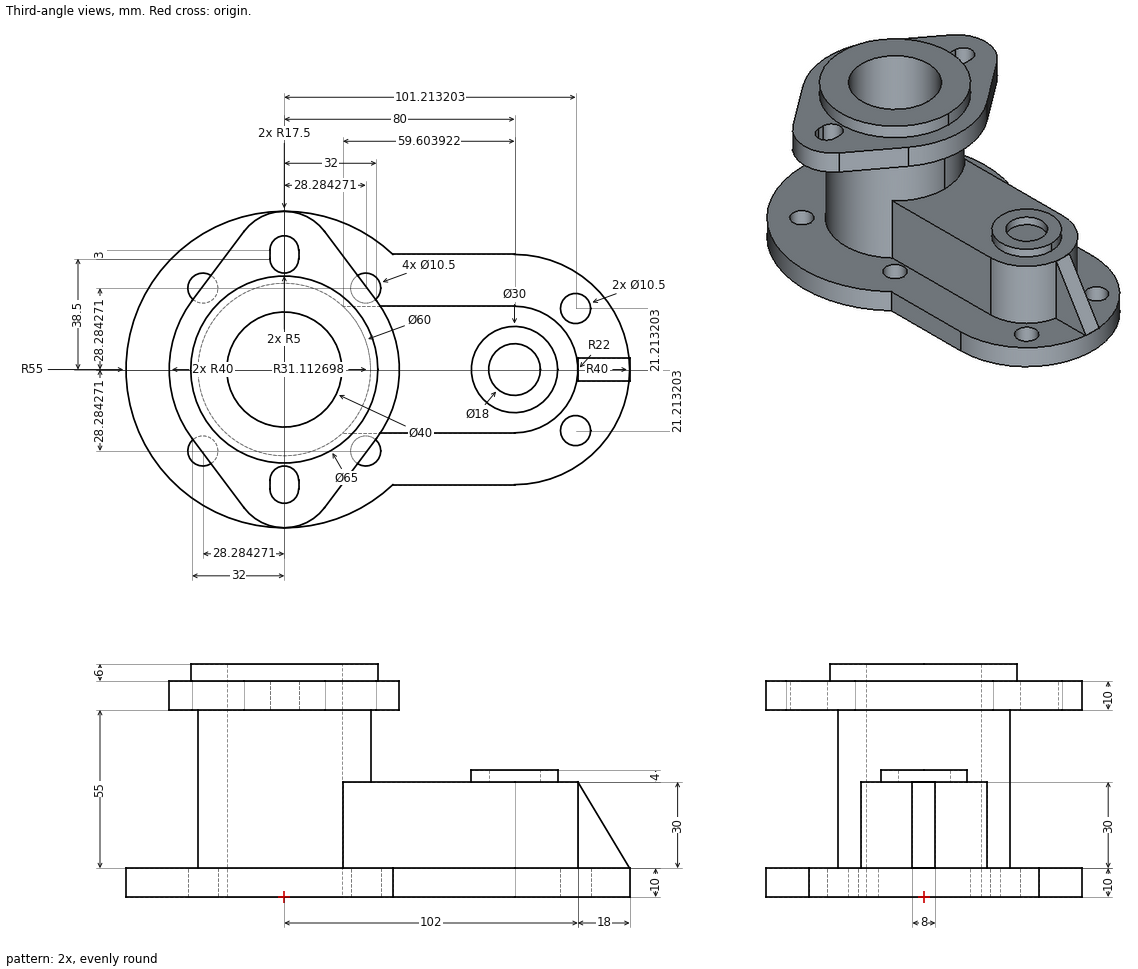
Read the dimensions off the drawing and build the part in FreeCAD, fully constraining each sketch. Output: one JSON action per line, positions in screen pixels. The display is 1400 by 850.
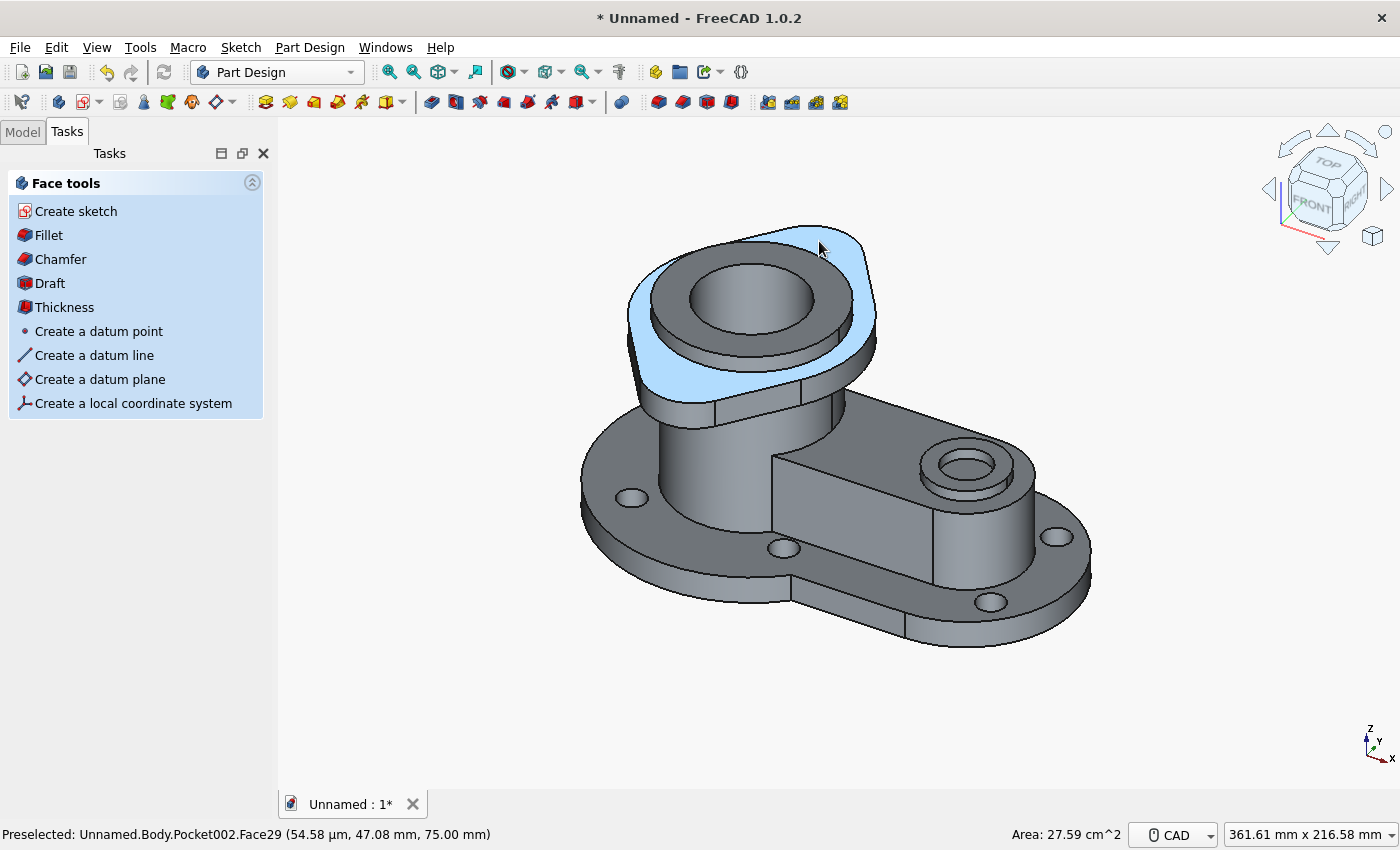
{"action": "left_click", "coordinate": [84, 102]}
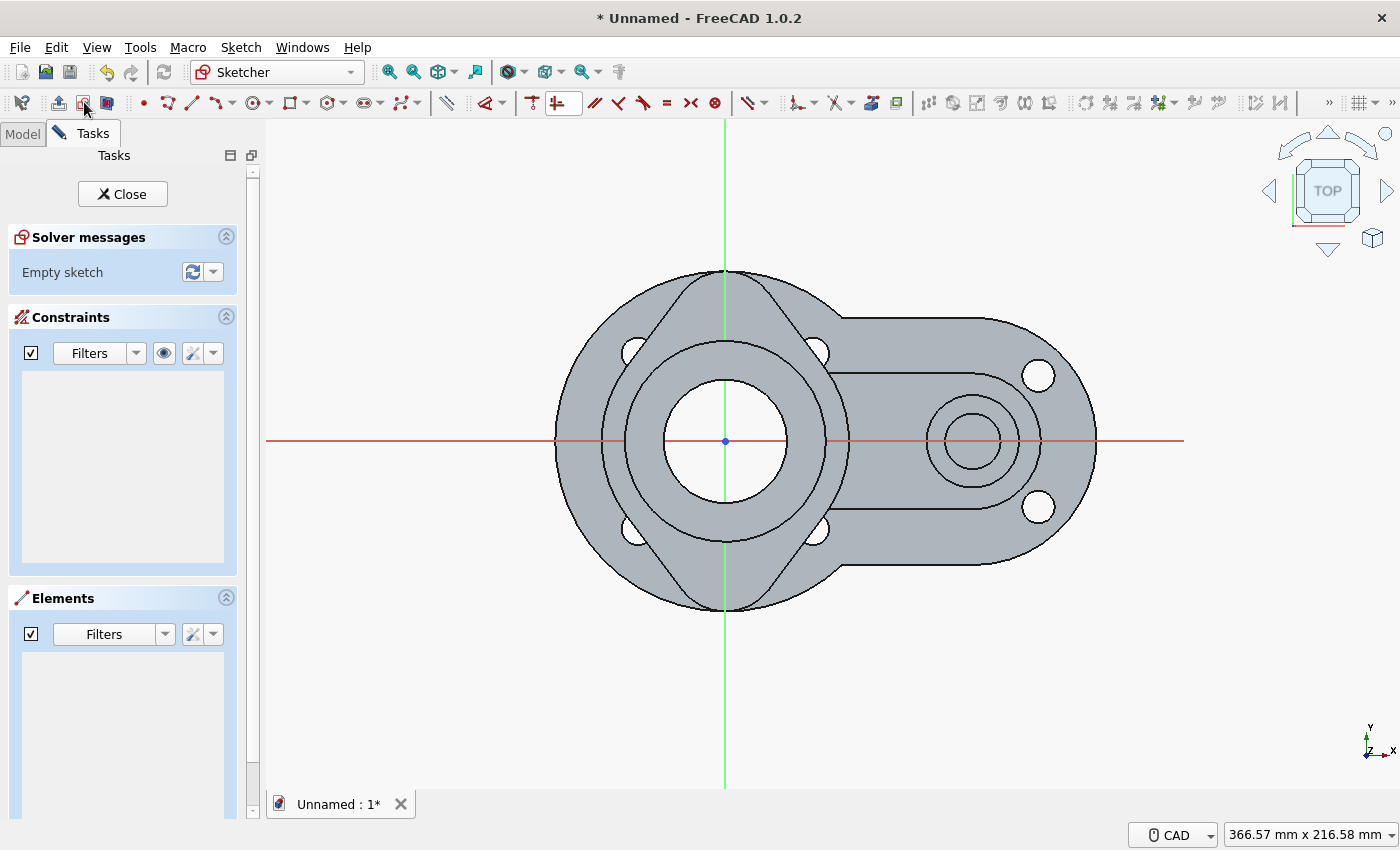
{"action": "key", "text": "q s"}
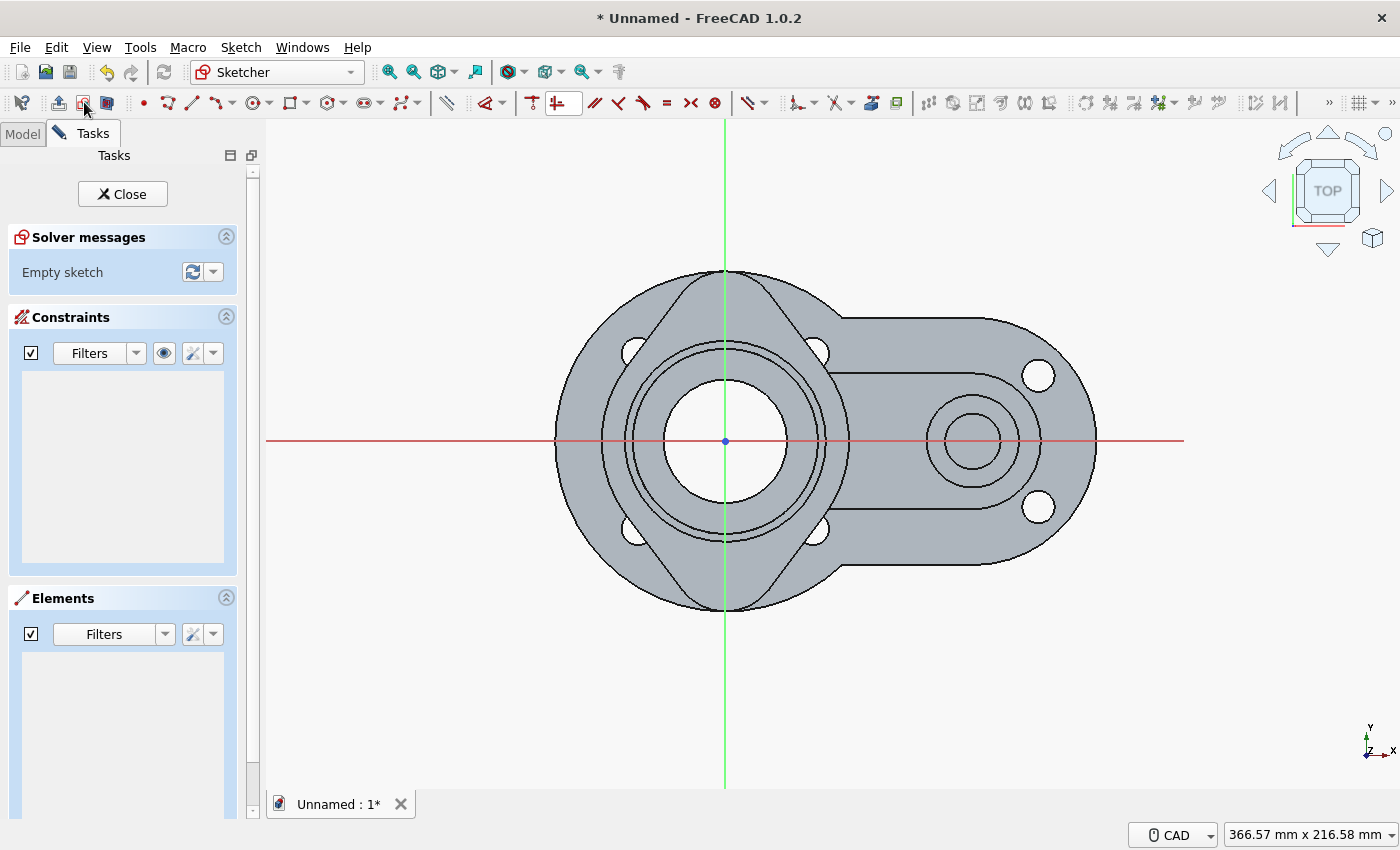
{"action": "scroll", "coordinate": [721, 304], "scroll_direction": "up", "scroll_amount": 12}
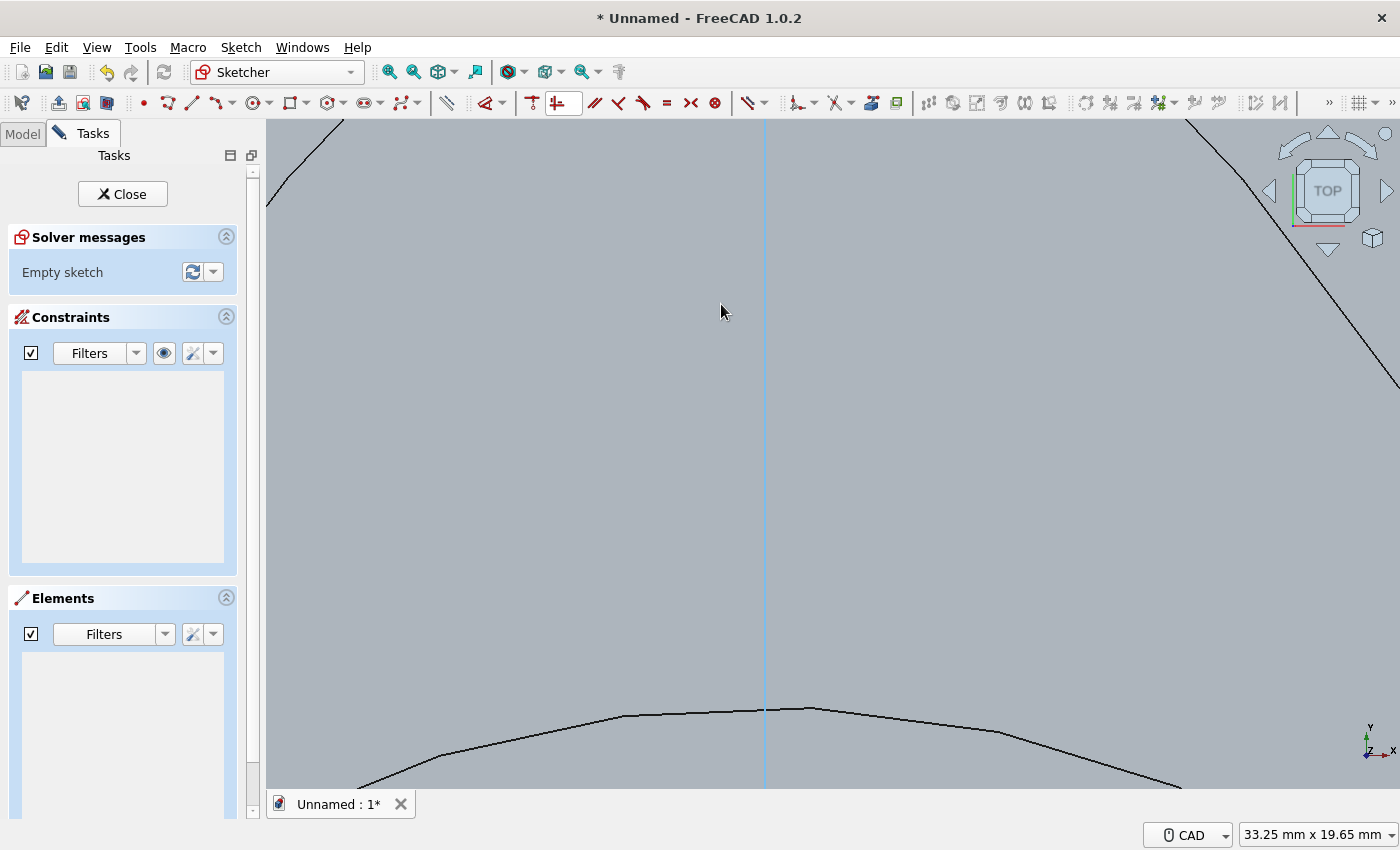
{"action": "key", "text": "g s"}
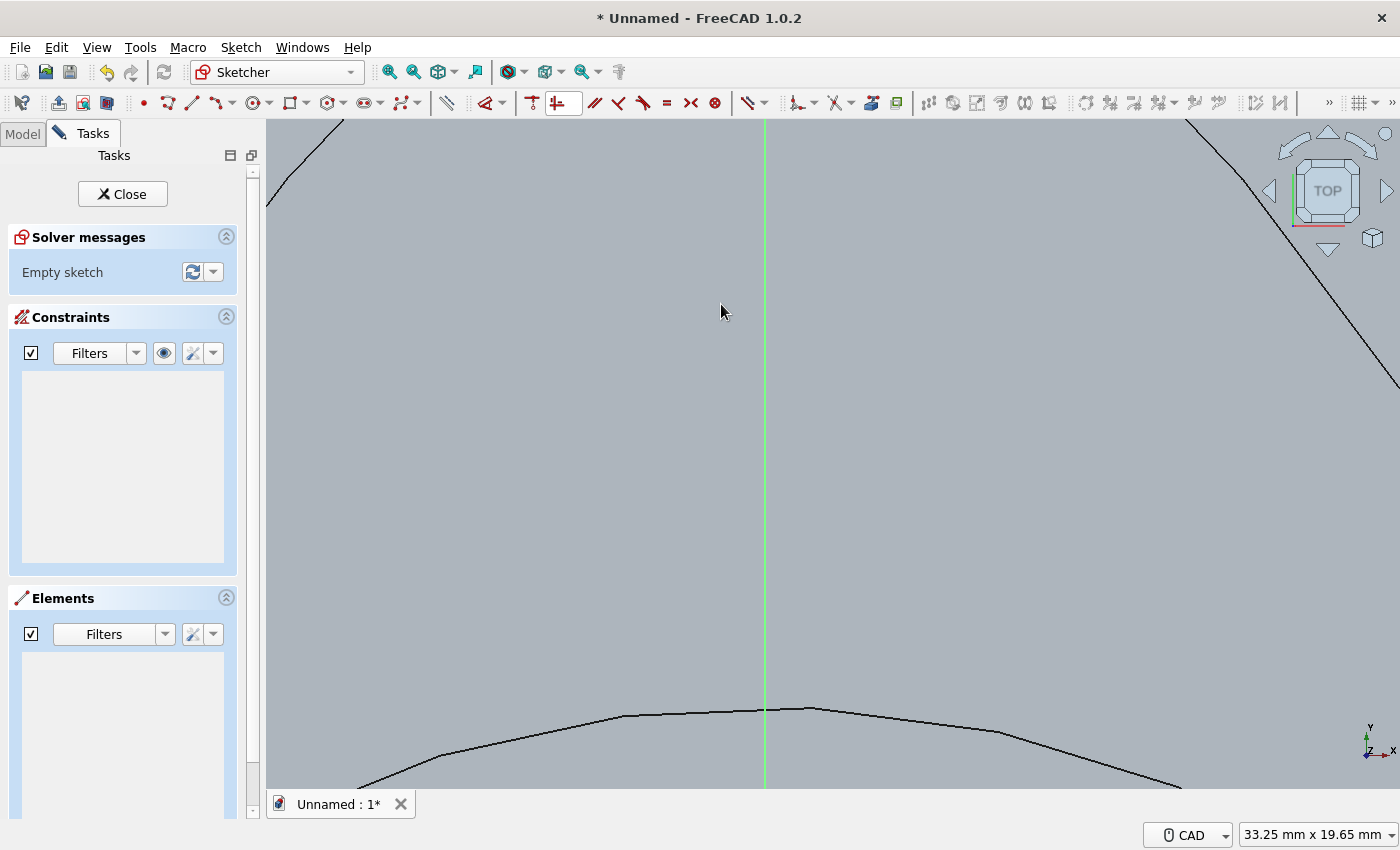
{"action": "left_click", "coordinate": [765, 503]}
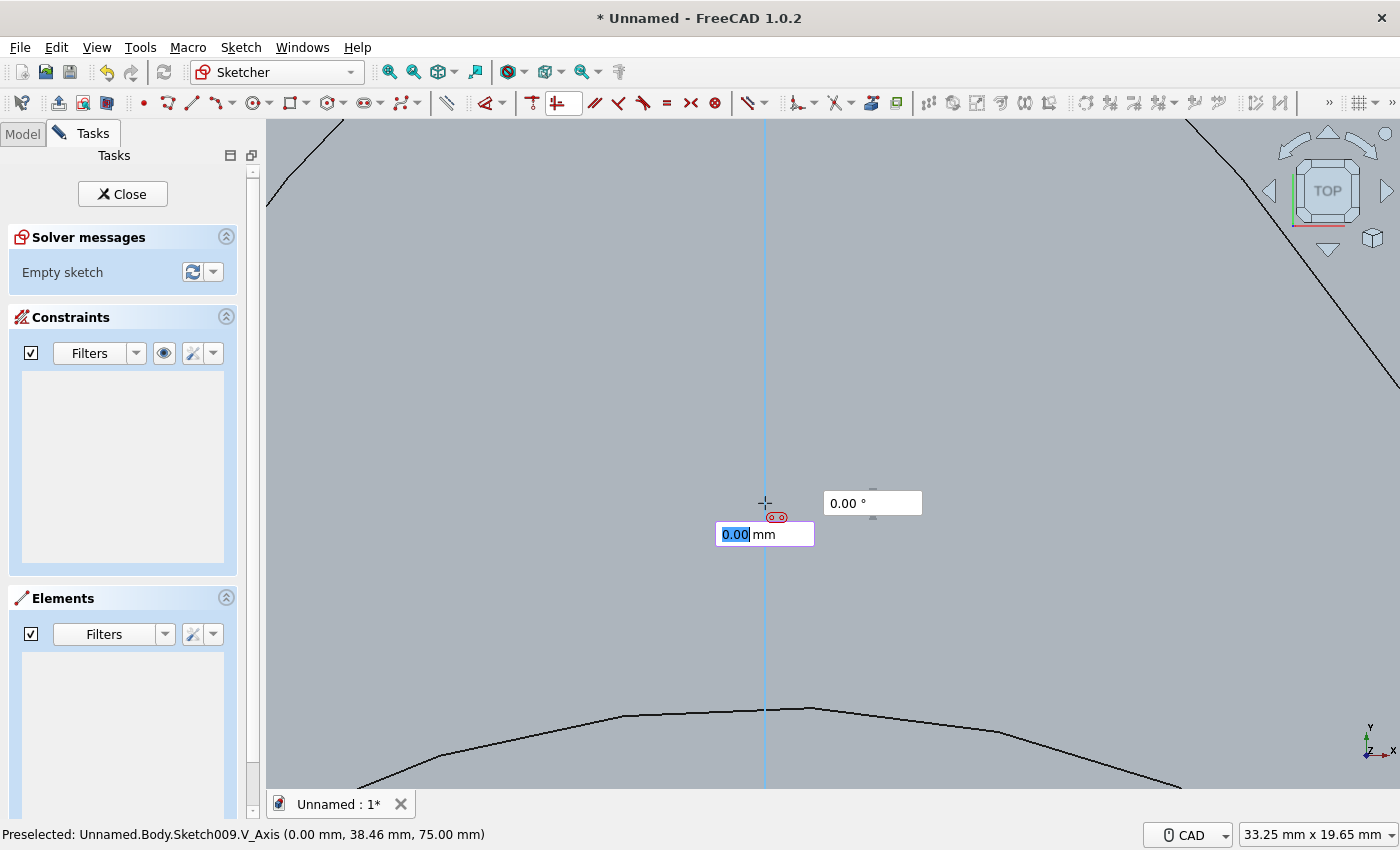
{"action": "left_click", "coordinate": [774, 400]}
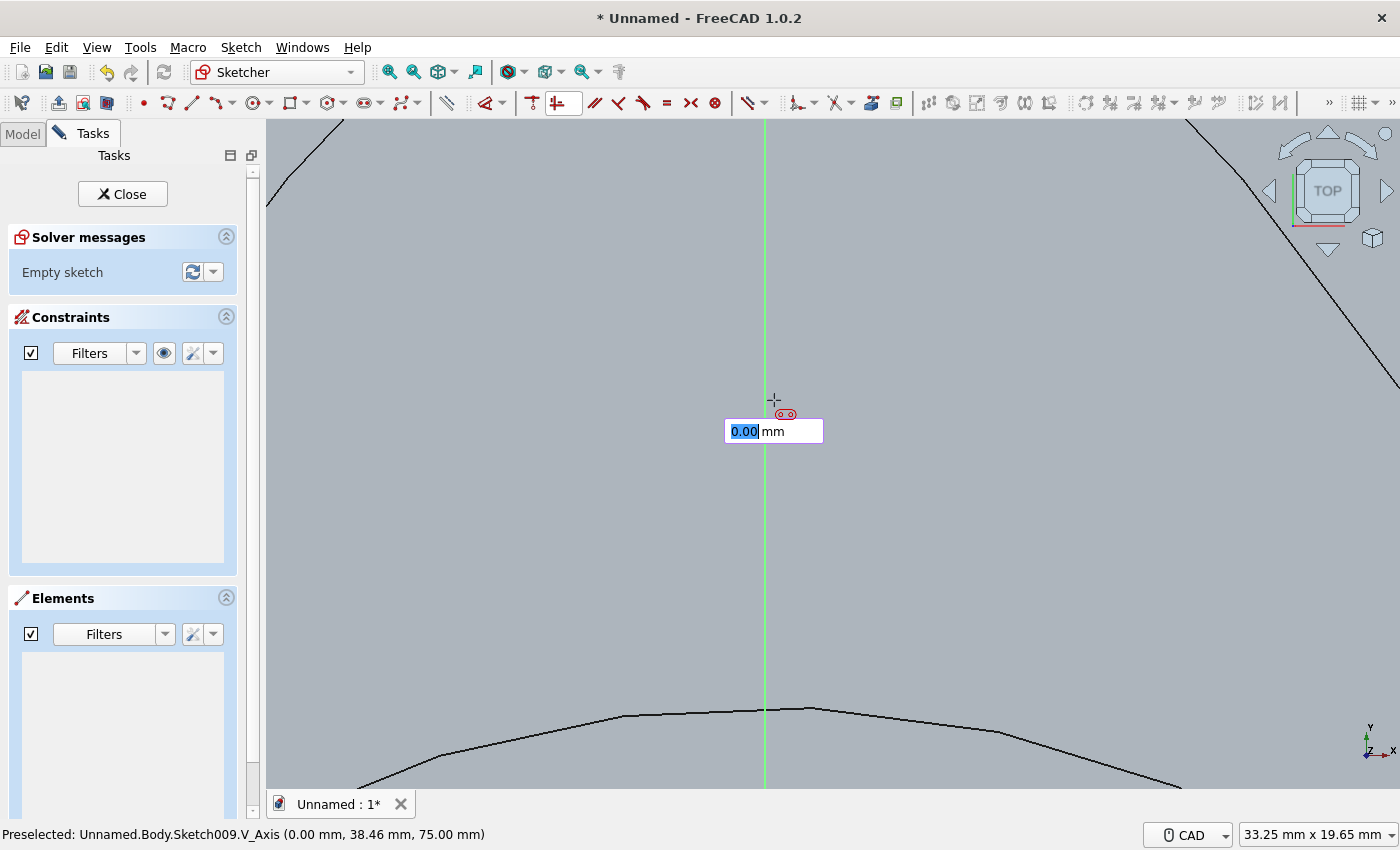
{"action": "left_click", "coordinate": [594, 451]}
{"action": "key", "text": "Escape"}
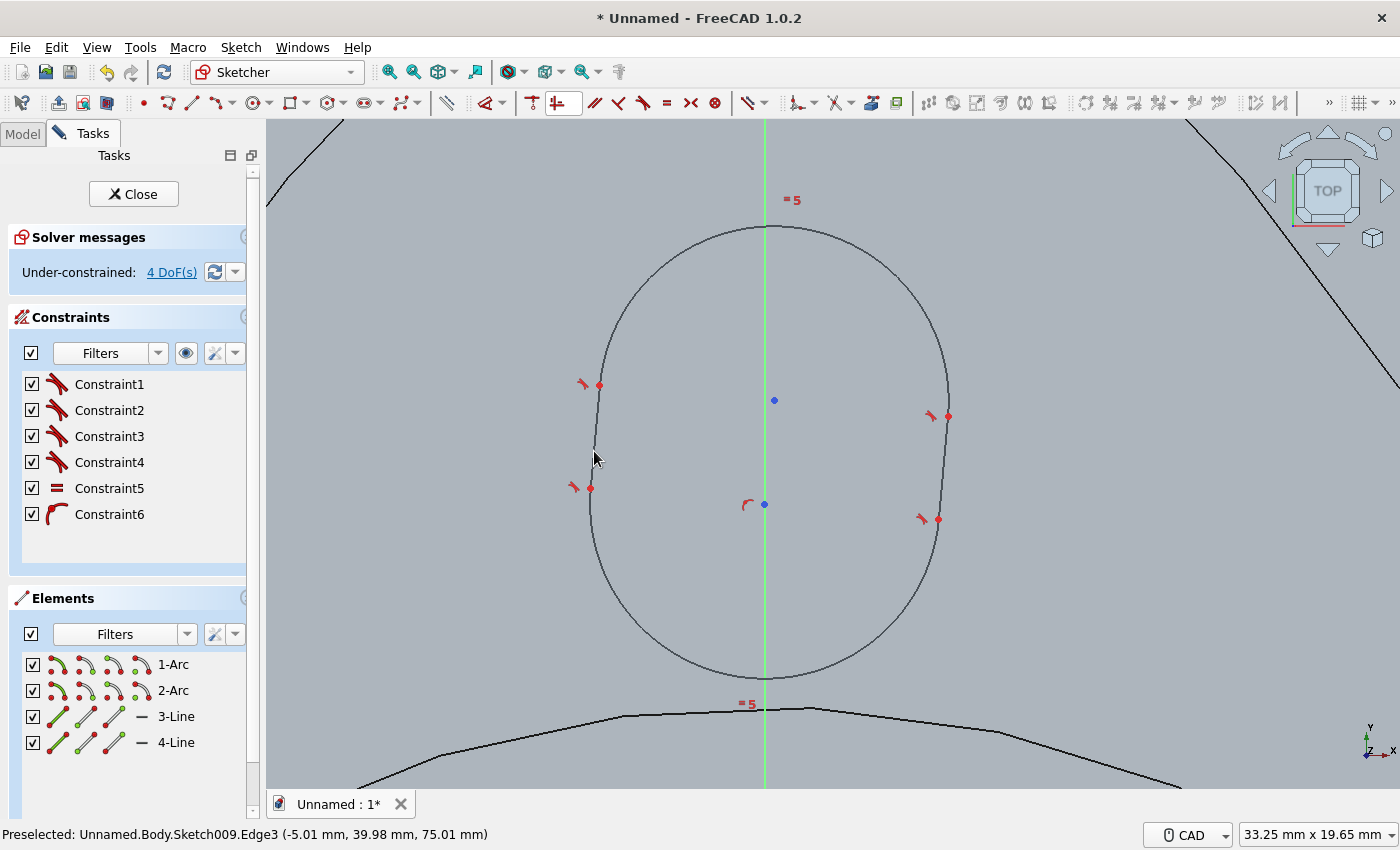
{"action": "left_click", "coordinate": [594, 458]}